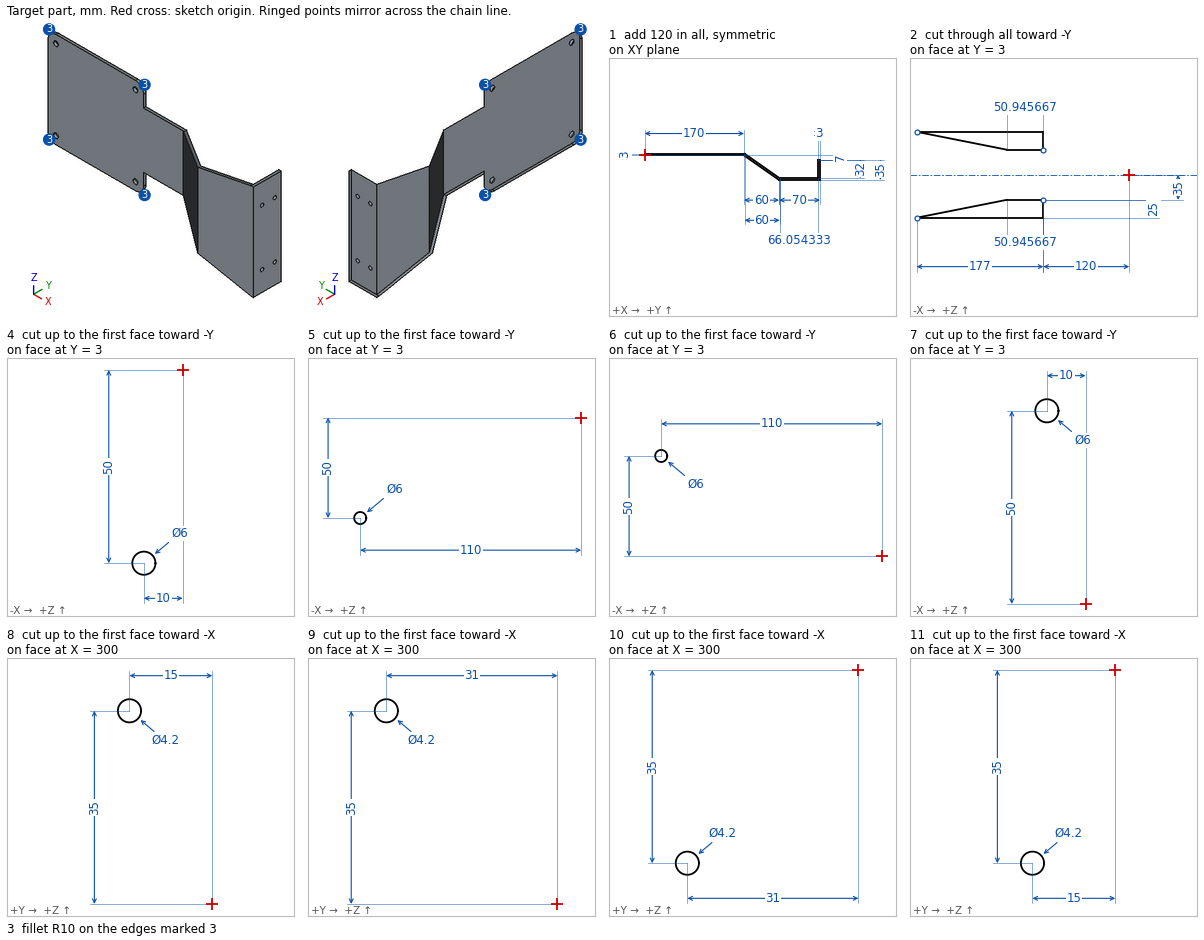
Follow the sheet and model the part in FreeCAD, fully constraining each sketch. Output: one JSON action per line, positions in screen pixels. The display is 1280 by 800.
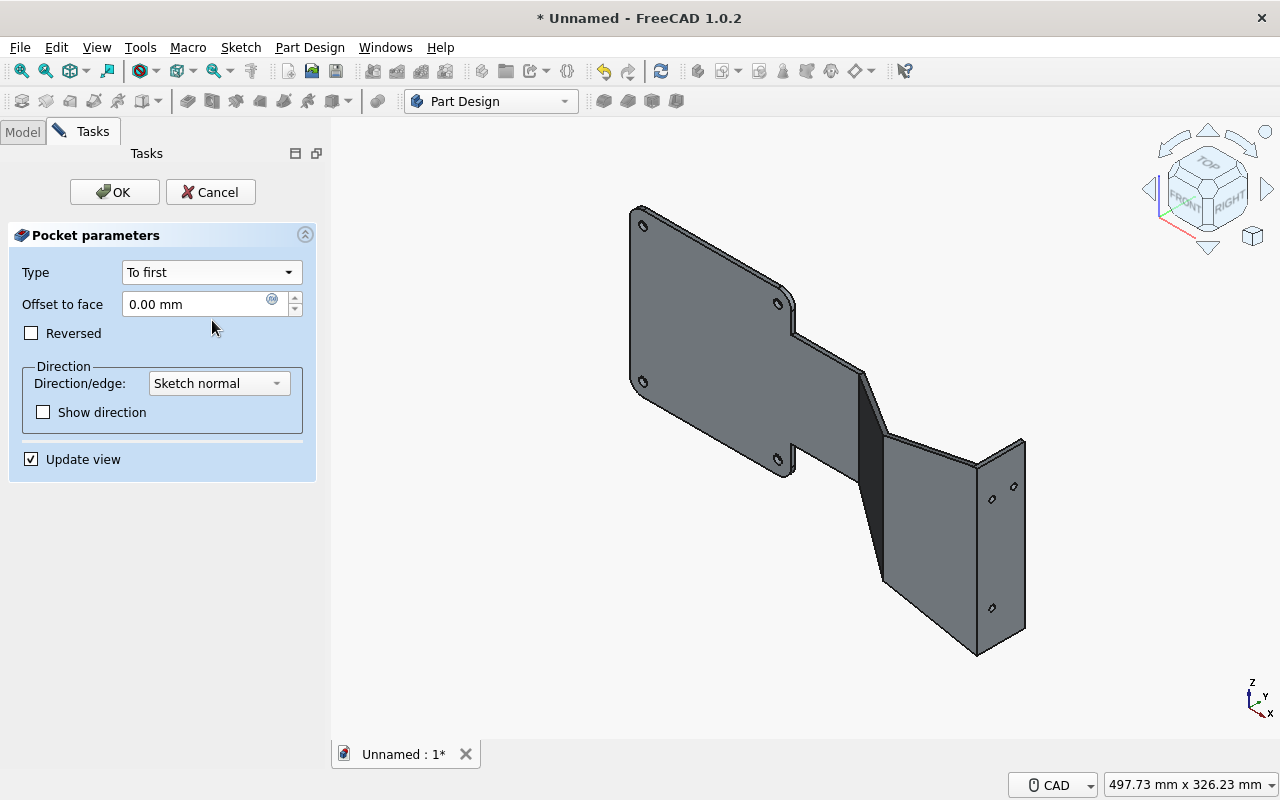
{"action": "left_click", "coordinate": [115, 192]}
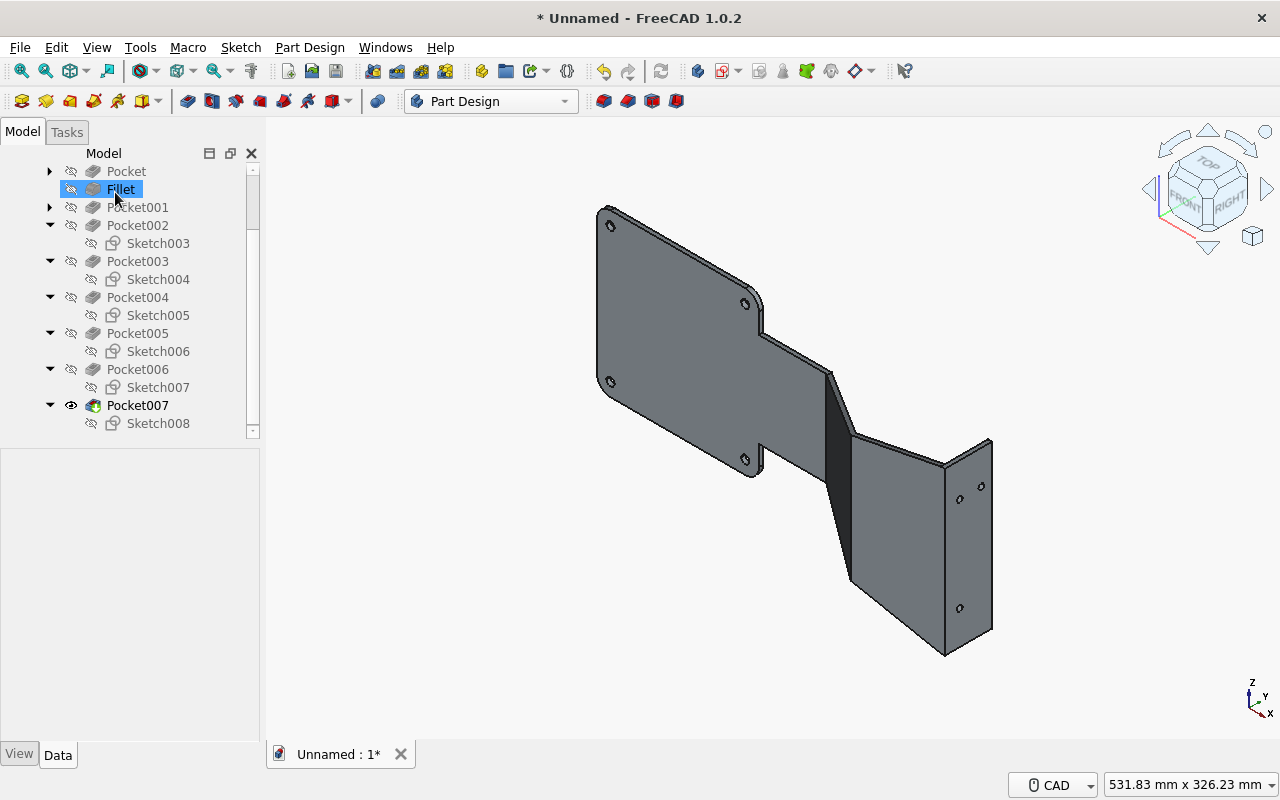
{"action": "left_click", "coordinate": [968, 548]}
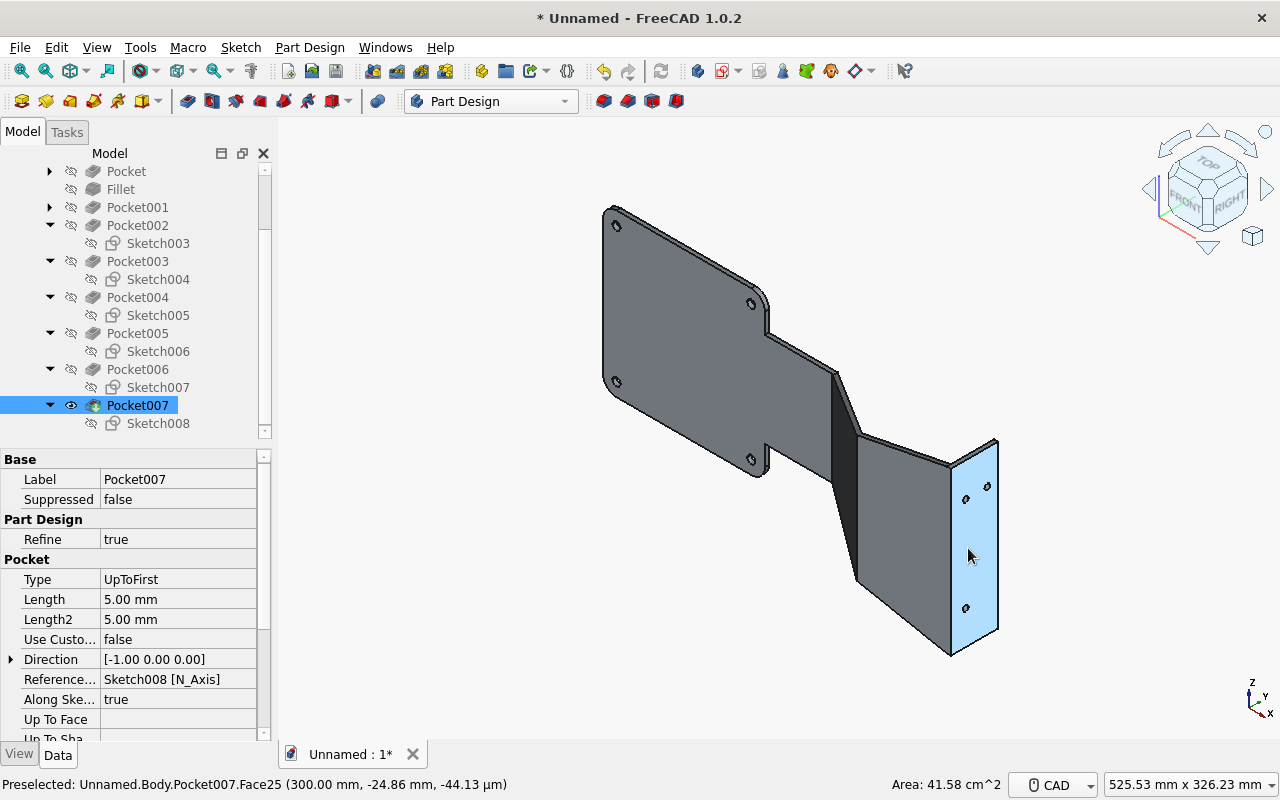
{"action": "left_click", "coordinate": [722, 72]}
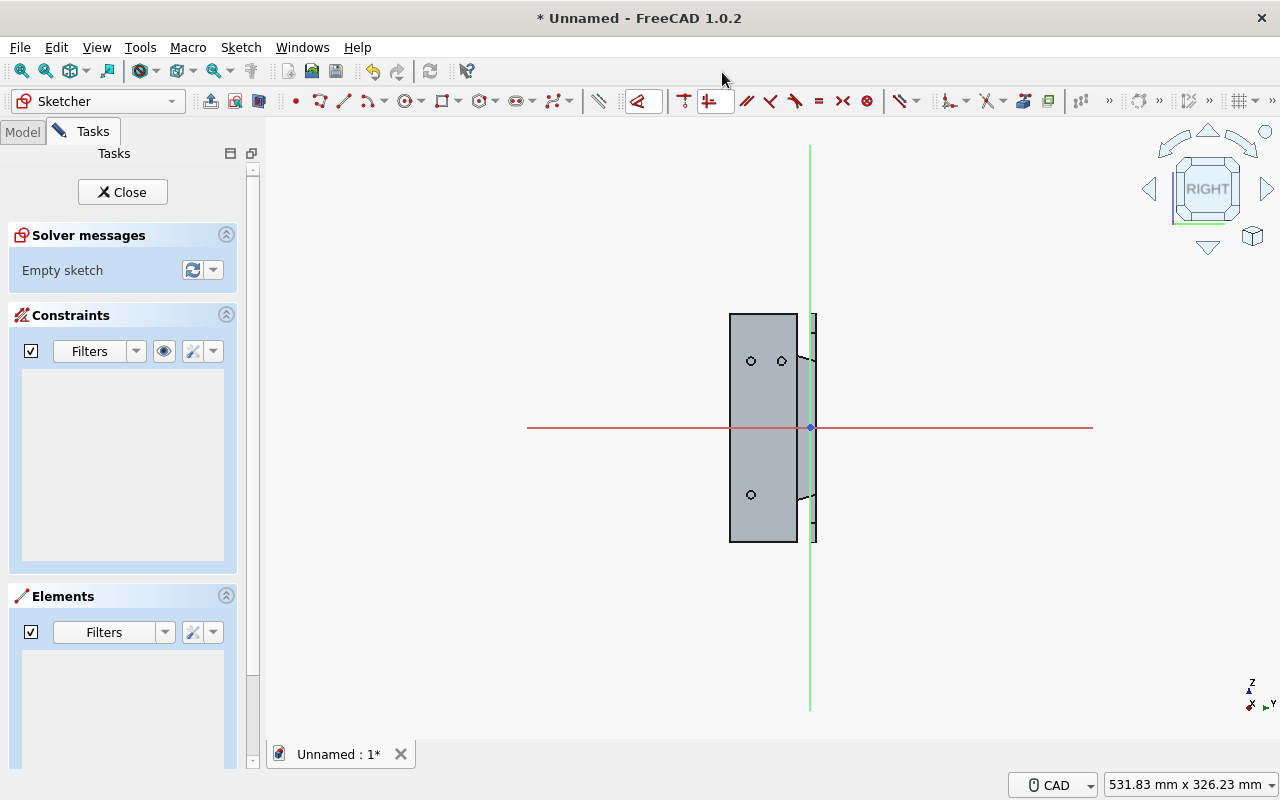
{"action": "scroll", "coordinate": [786, 498], "scroll_direction": "up", "scroll_amount": 15}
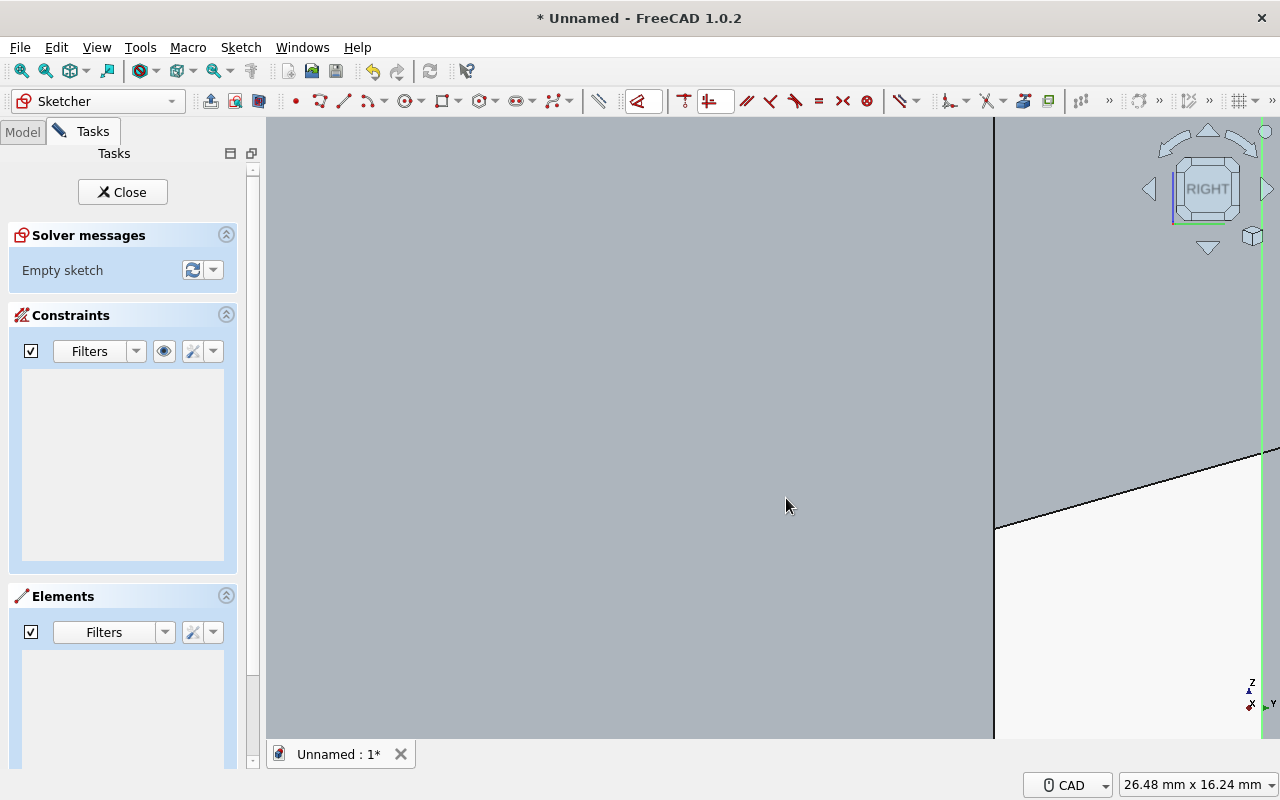
{"action": "scroll", "coordinate": [677, 416], "scroll_direction": "up", "scroll_amount": 5}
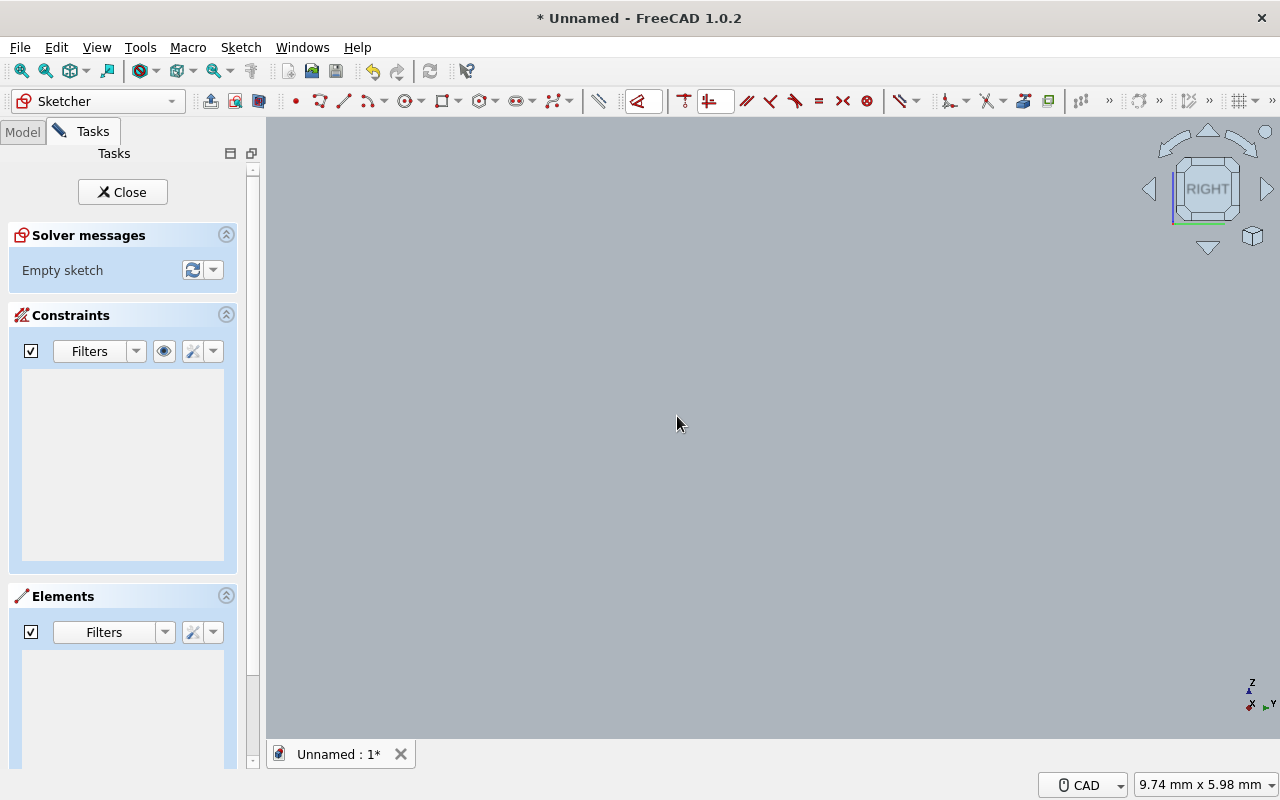
{"action": "left_click", "coordinate": [406, 102]}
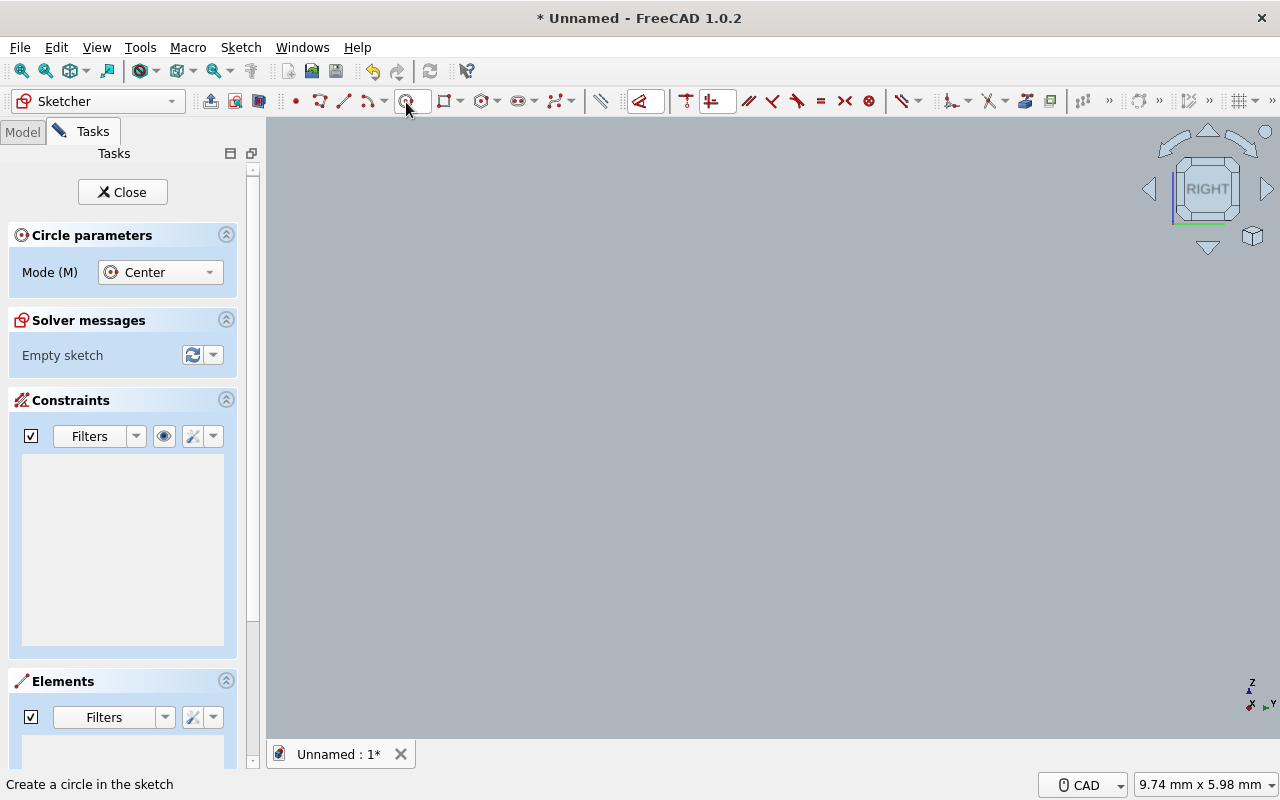
{"action": "left_click", "coordinate": [705, 428]}
{"action": "left_click", "coordinate": [859, 273]}
{"action": "key", "text": "Escape"}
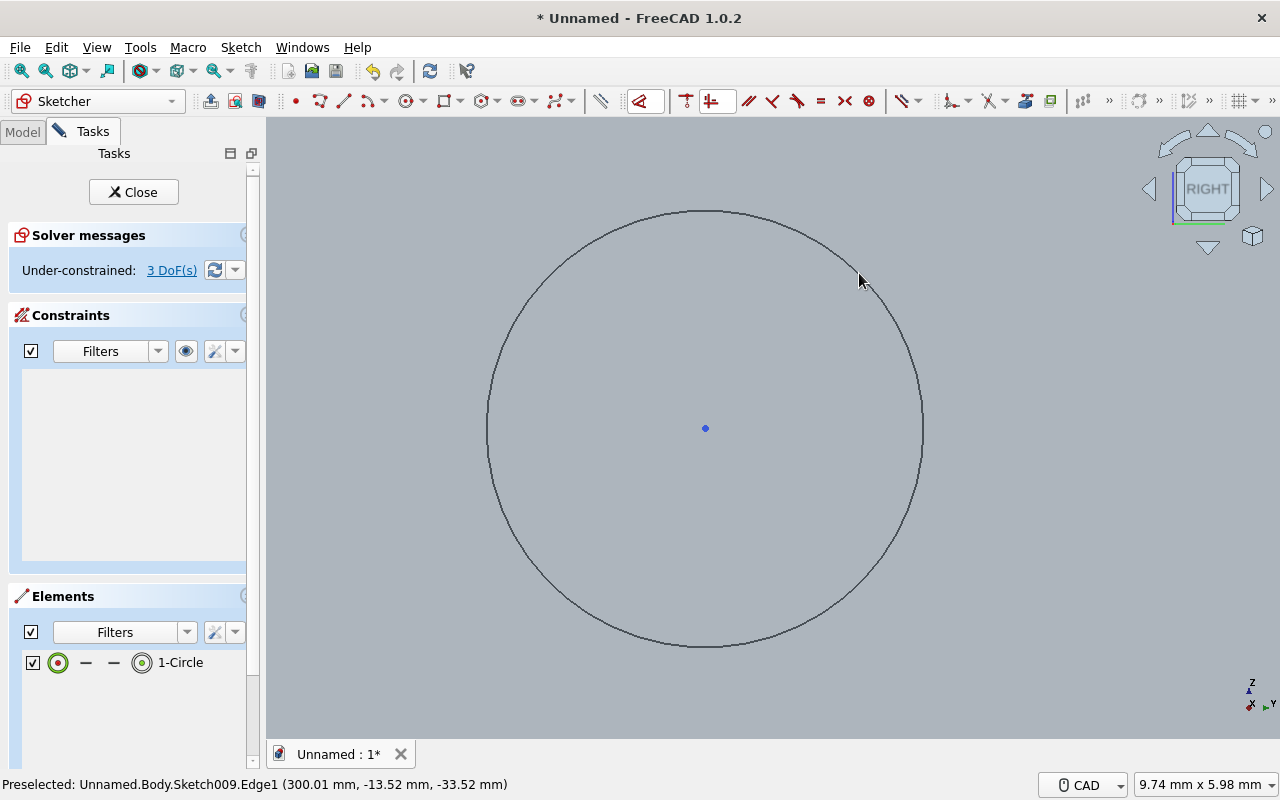
{"action": "left_click", "coordinate": [859, 274]}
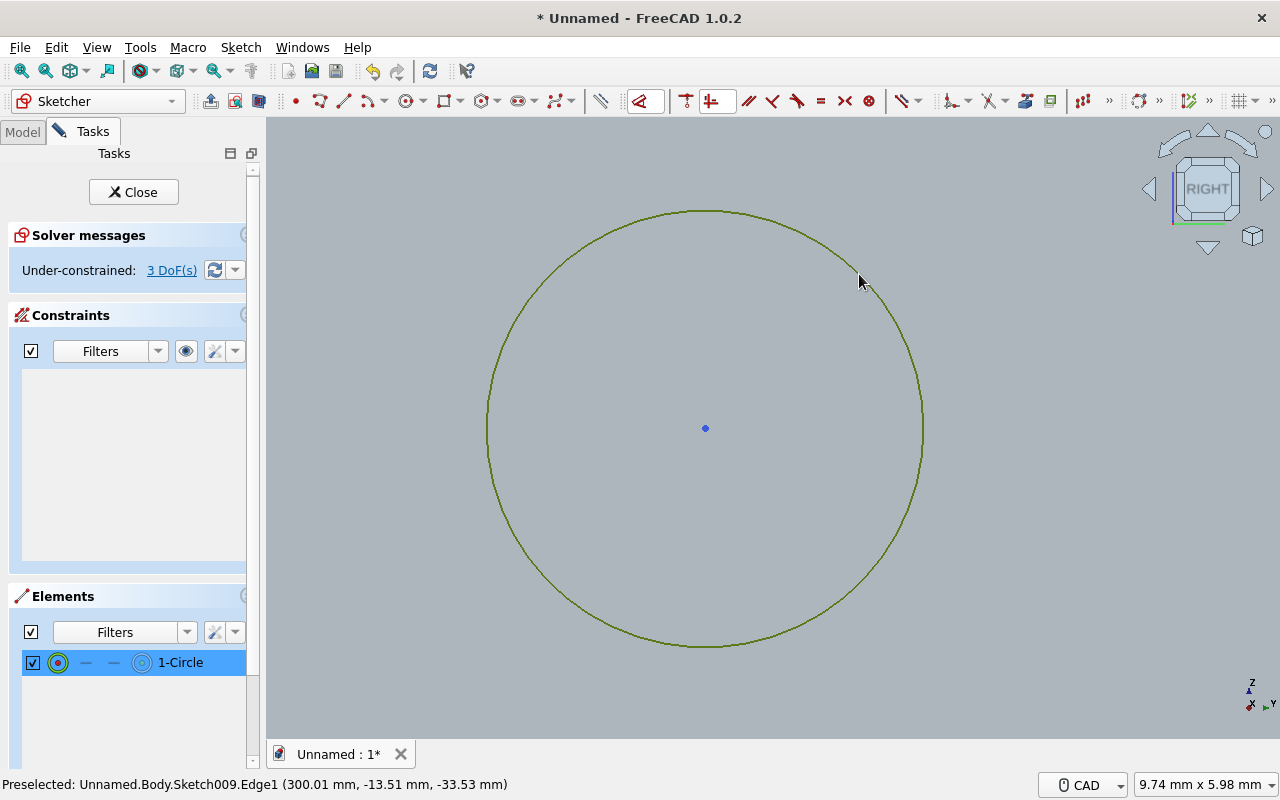
{"action": "left_click", "coordinate": [658, 102]}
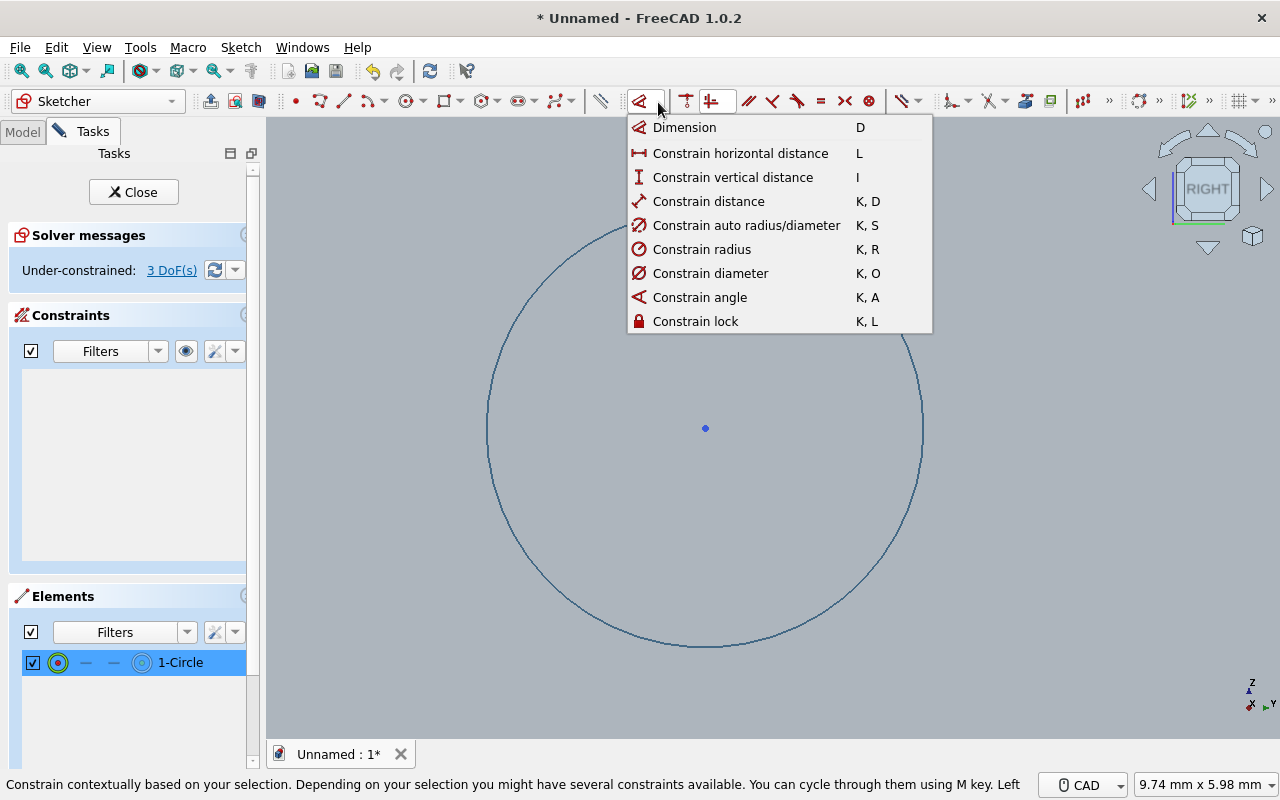
{"action": "left_click", "coordinate": [780, 273]}